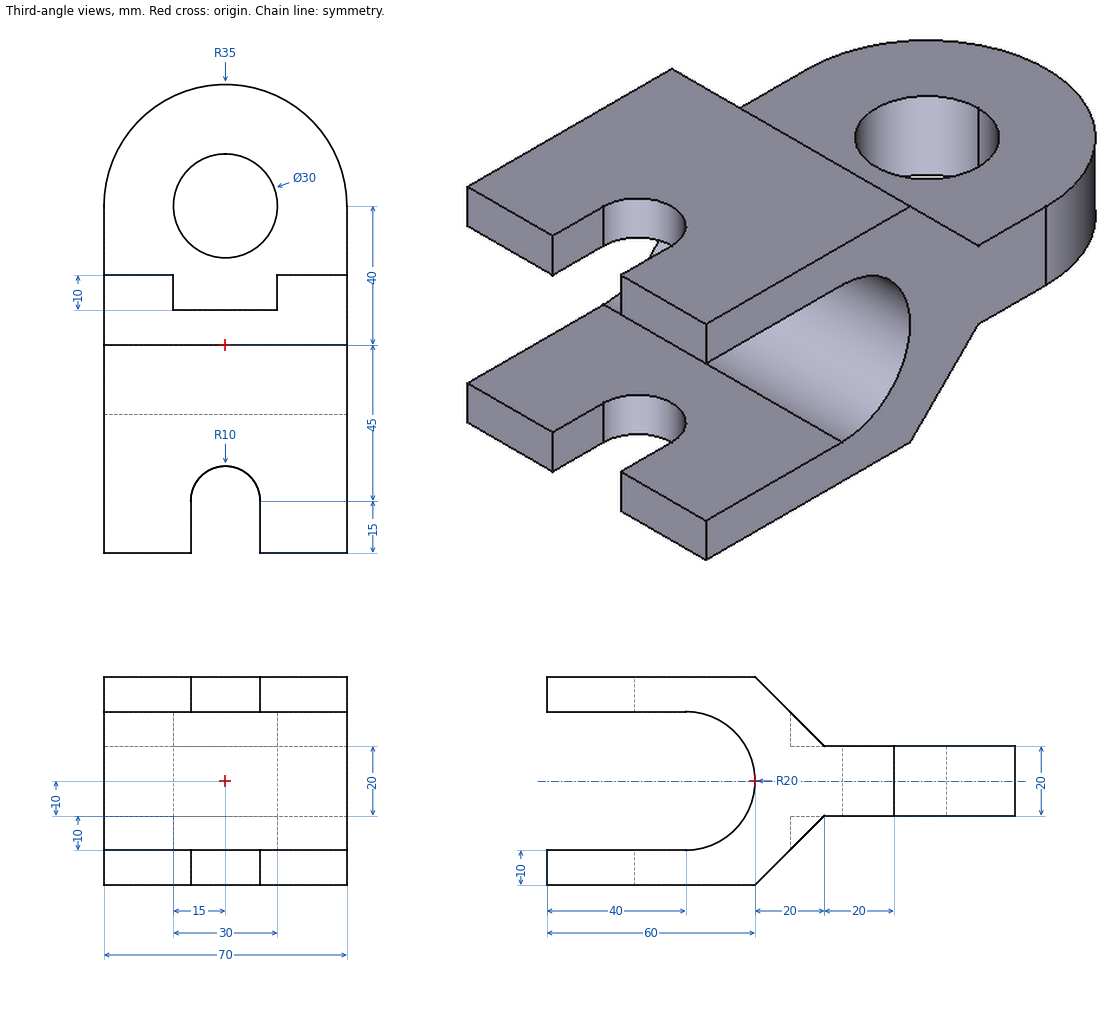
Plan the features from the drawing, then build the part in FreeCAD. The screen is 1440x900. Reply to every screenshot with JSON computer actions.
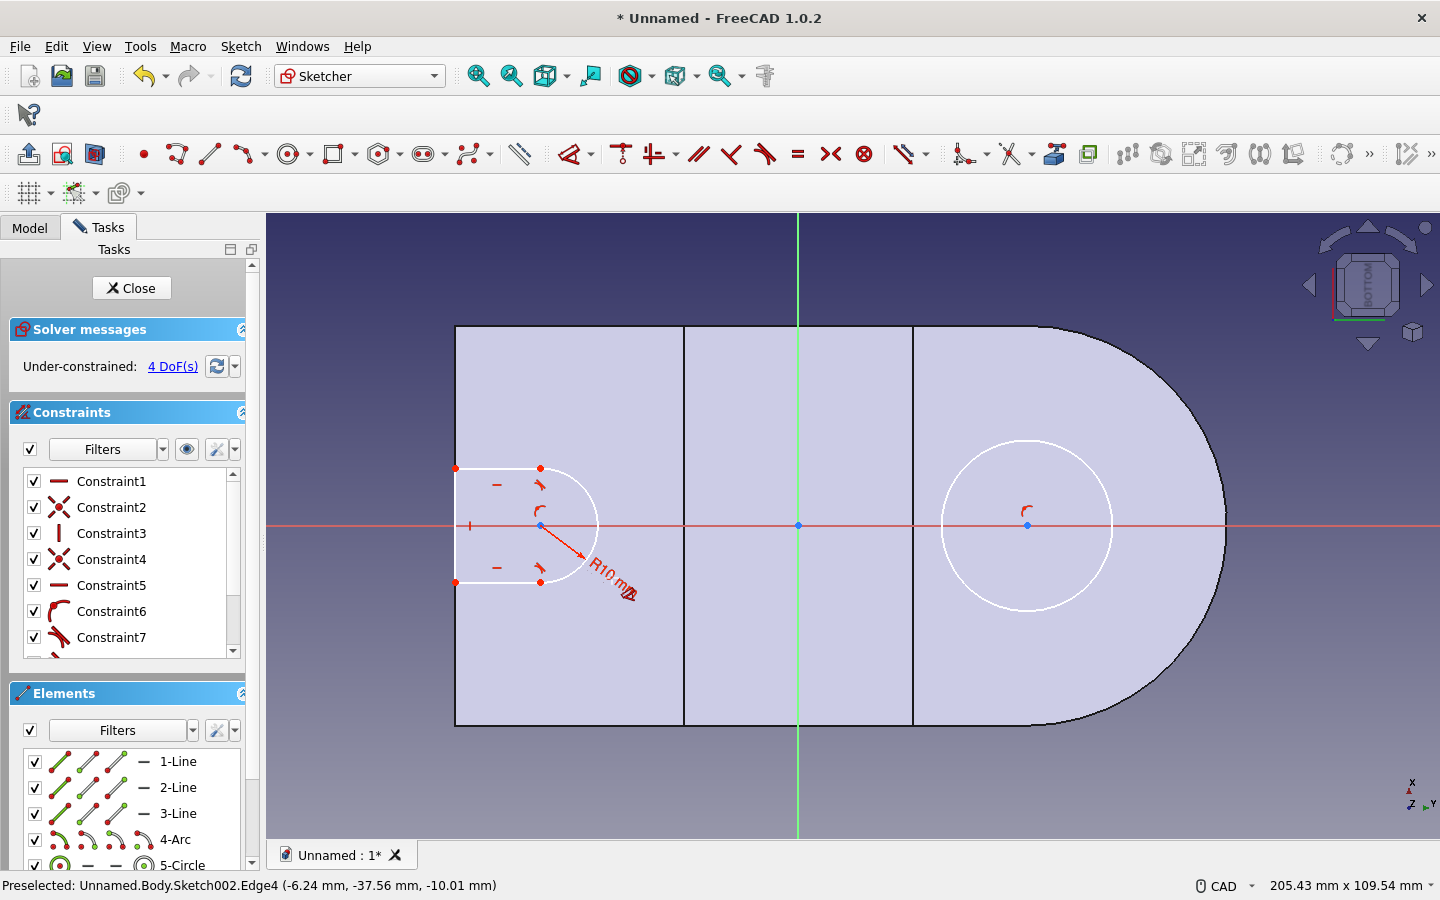
{"action": "left_click", "coordinate": [1087, 465]}
{"action": "left_click", "coordinate": [1109, 442]}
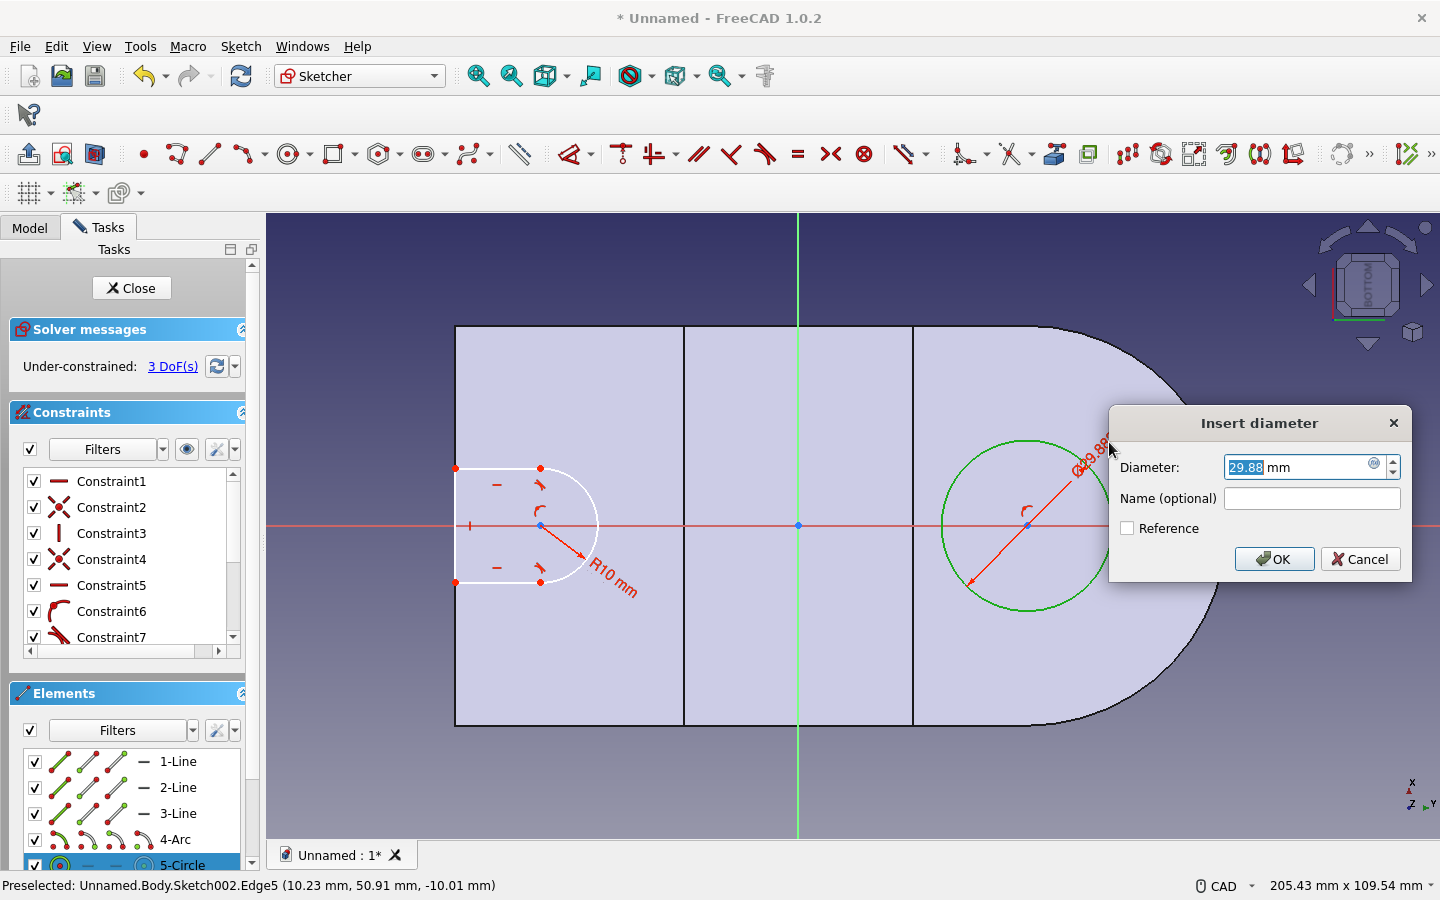
{"action": "type", "text": "30"}
{"action": "key", "text": "Return"}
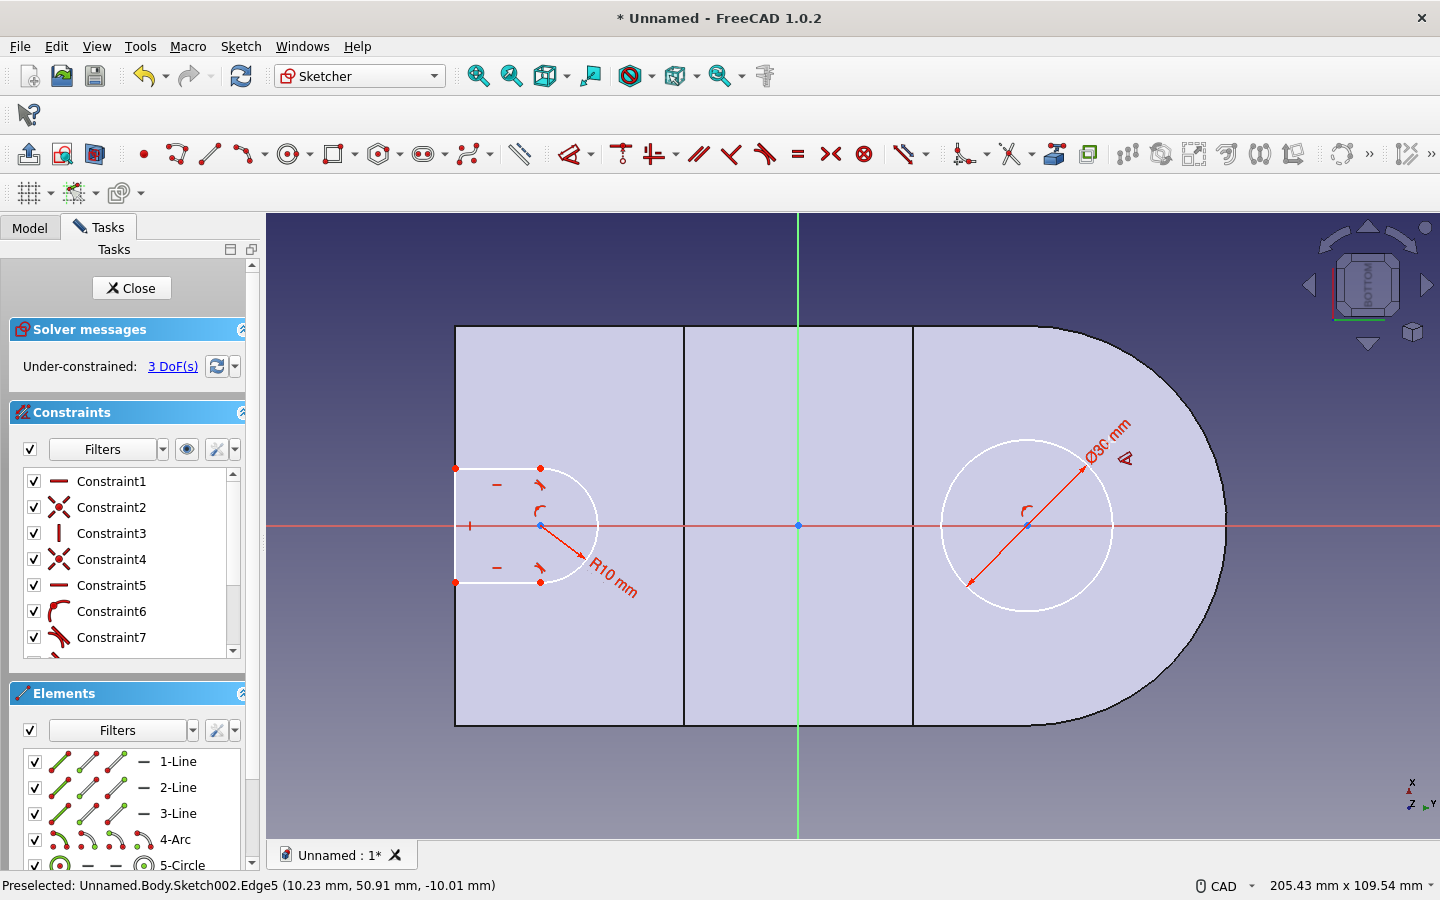
{"action": "left_click", "coordinate": [515, 469]}
{"action": "left_click", "coordinate": [498, 435]}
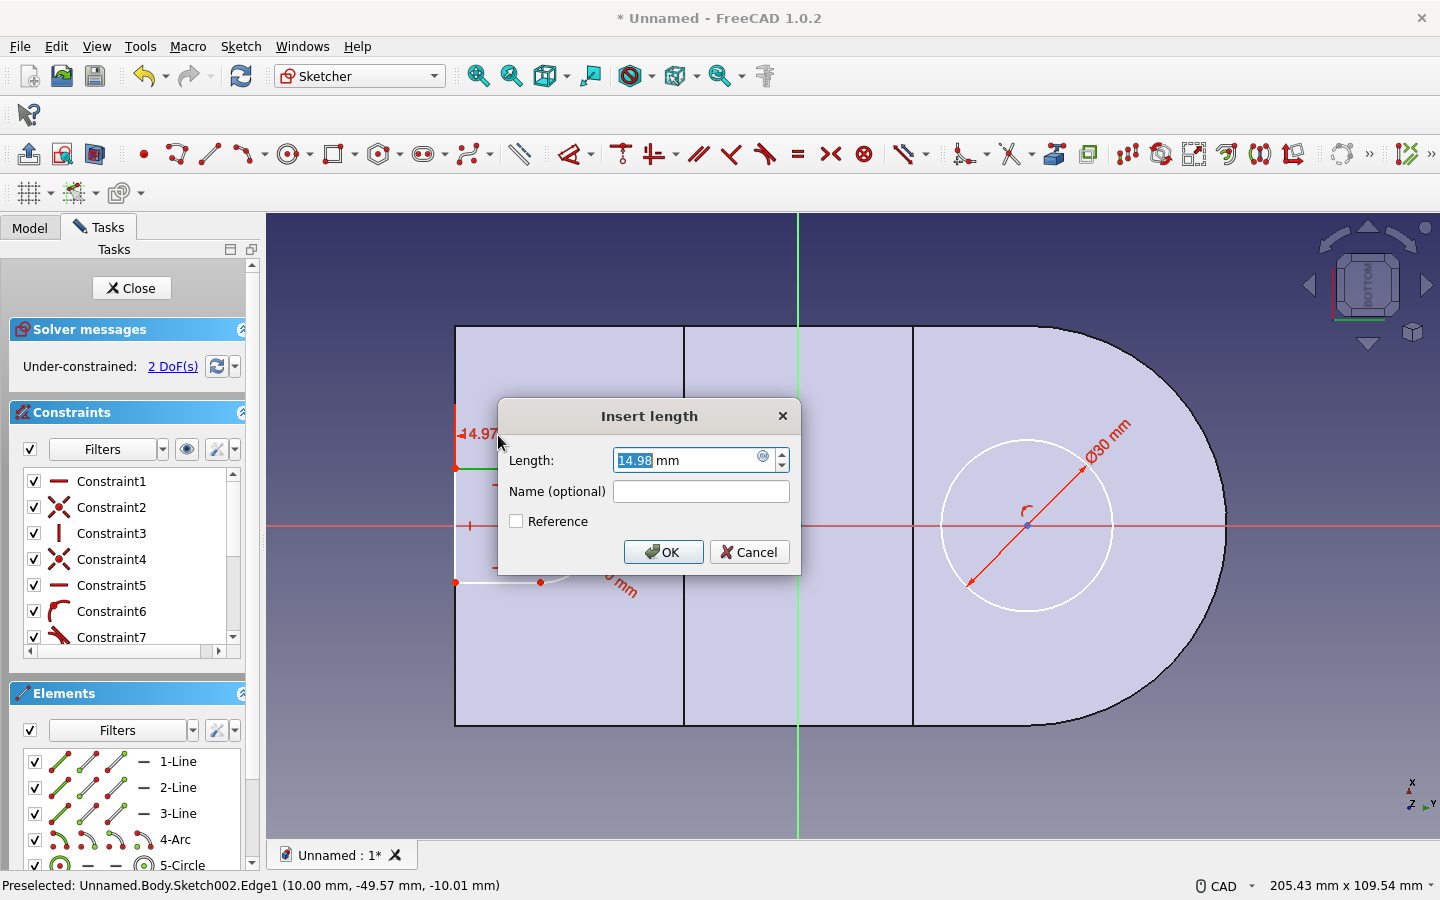
{"action": "type", "text": "15"}
{"action": "key", "text": "Return"}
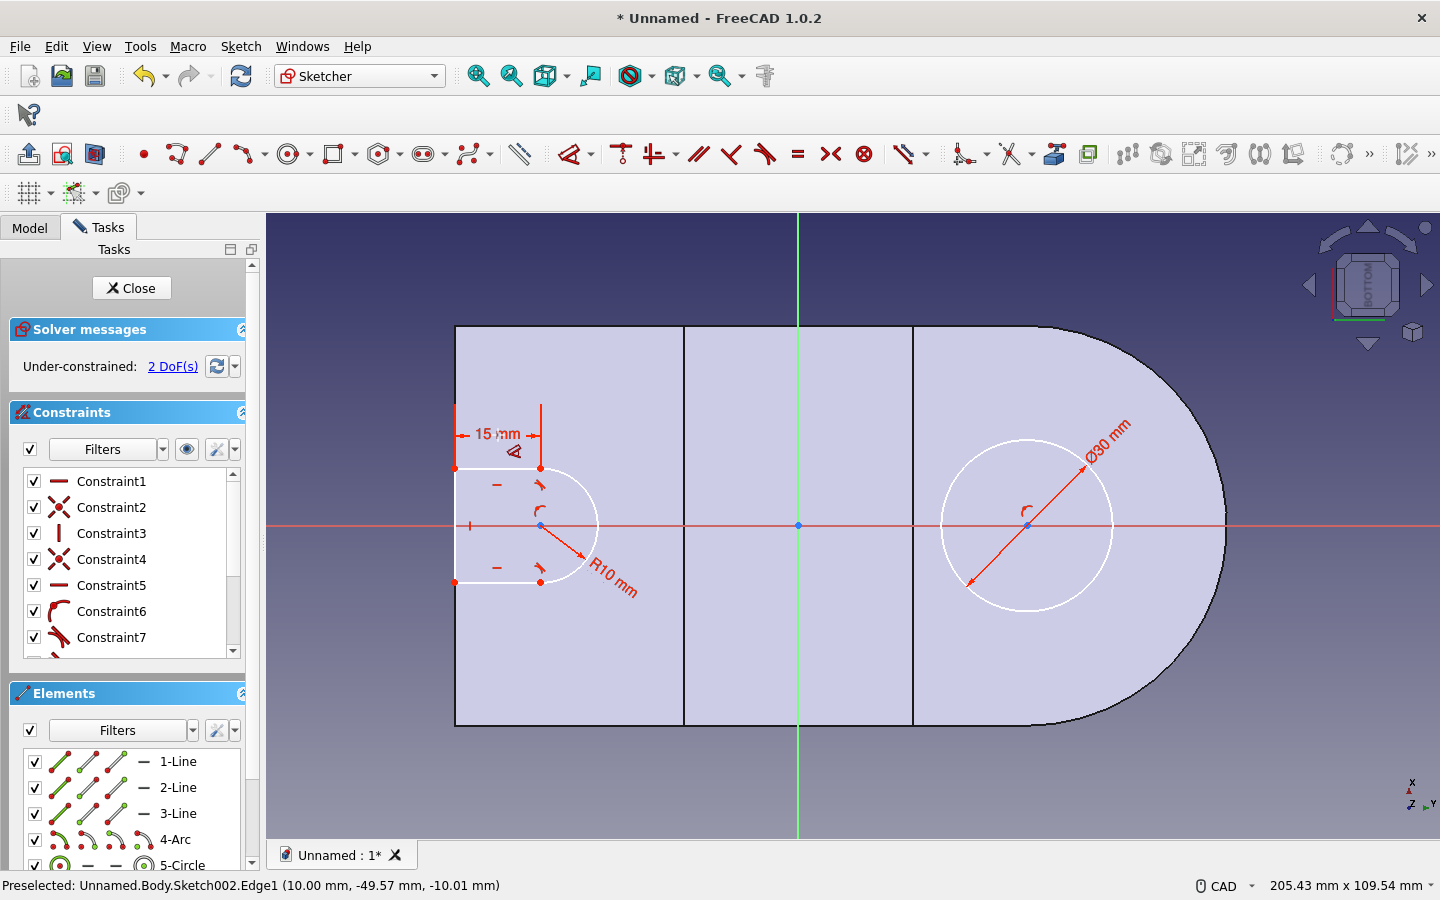
{"action": "left_click", "coordinate": [1027, 526]}
{"action": "left_click", "coordinate": [913, 560]}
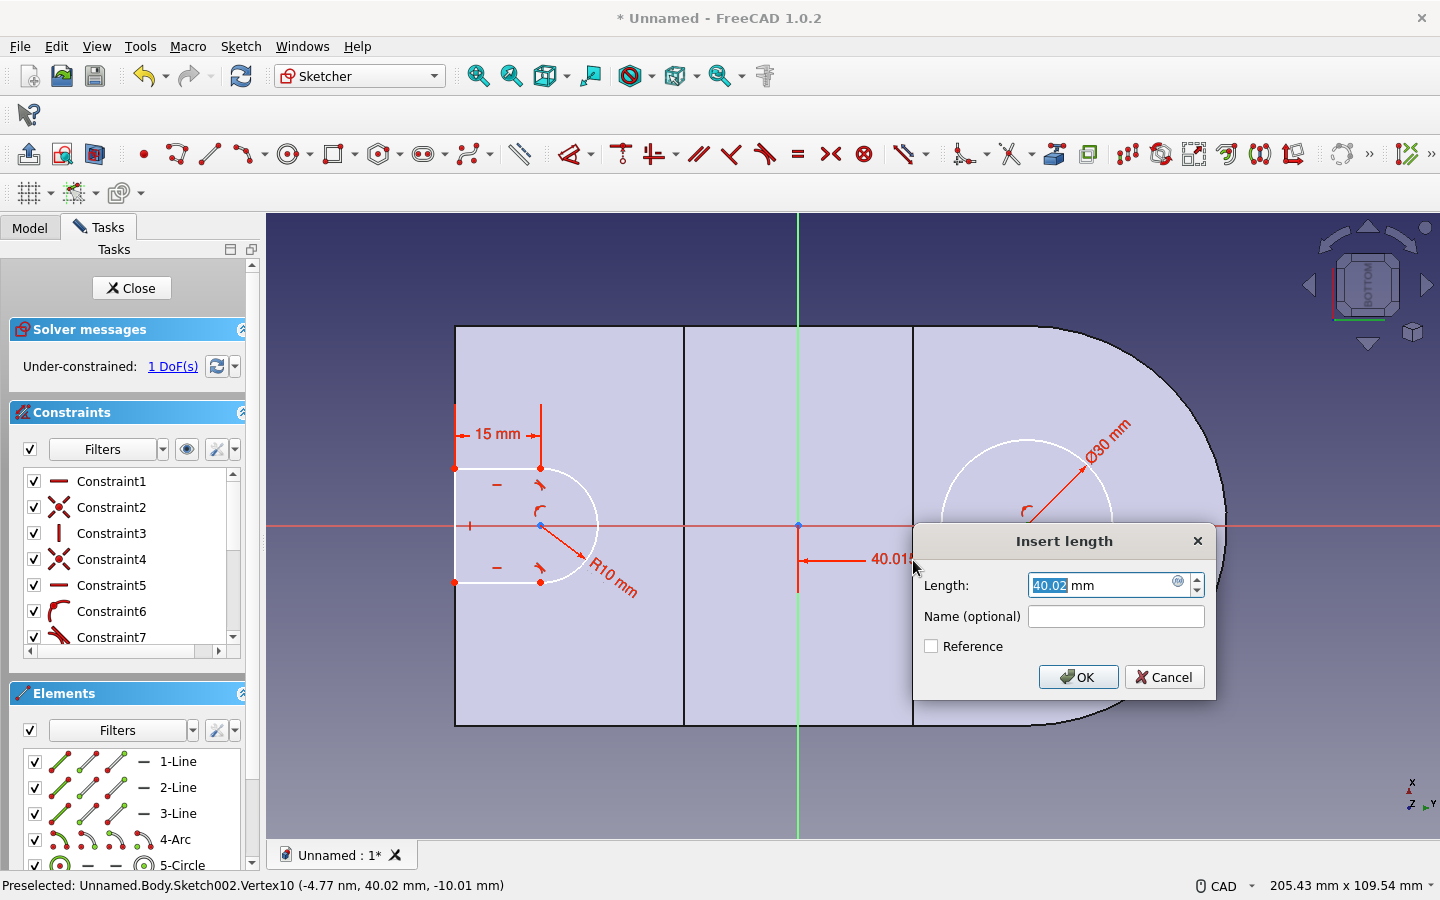
{"action": "type", "text": "40"}
{"action": "key", "text": "Return"}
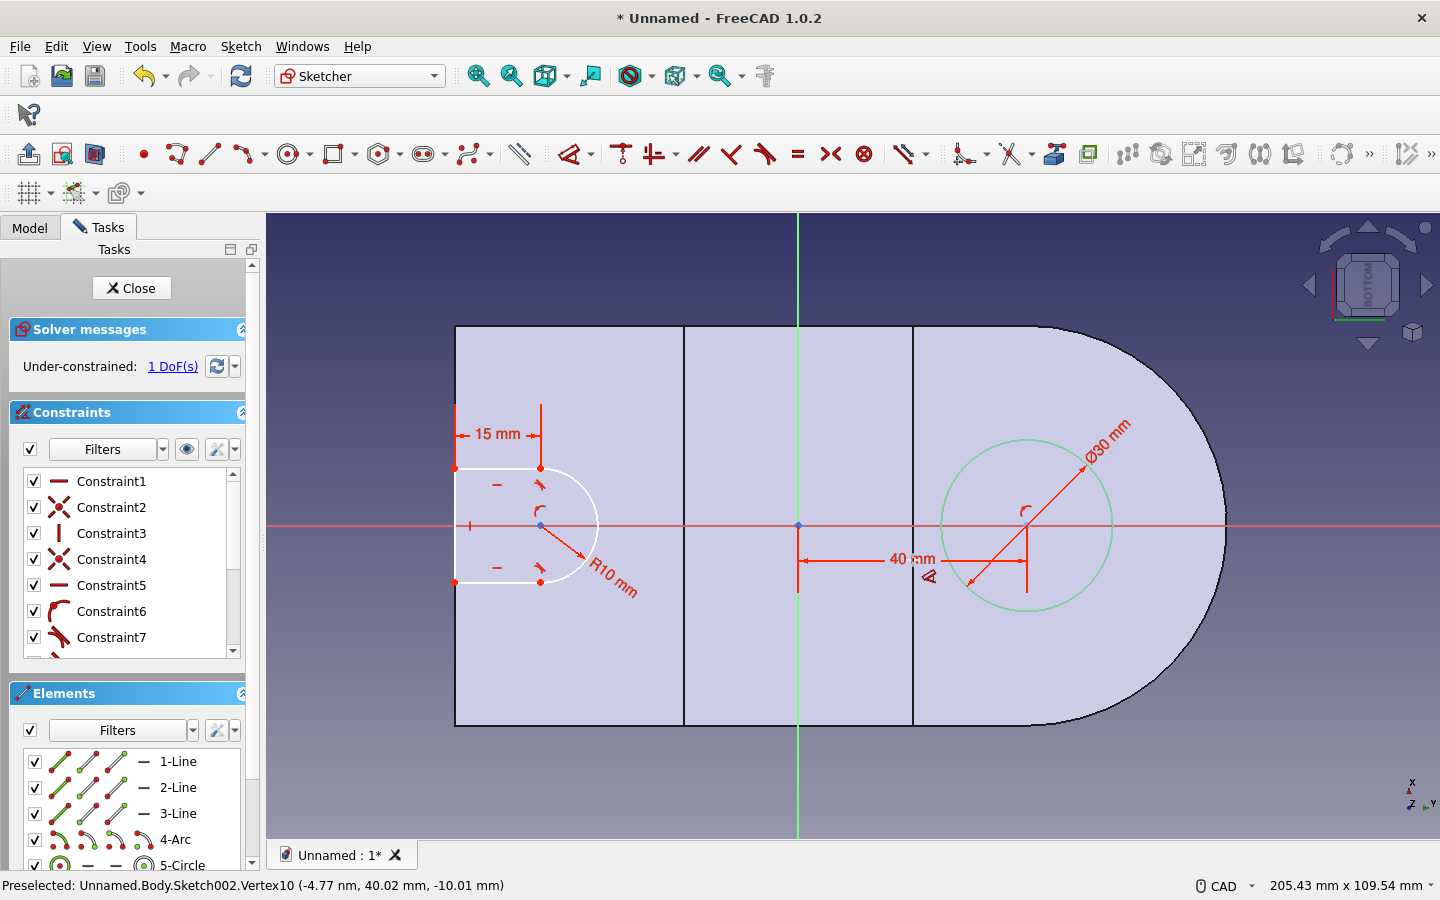
{"action": "left_click", "coordinate": [541, 469]}
{"action": "left_click", "coordinate": [669, 435]}